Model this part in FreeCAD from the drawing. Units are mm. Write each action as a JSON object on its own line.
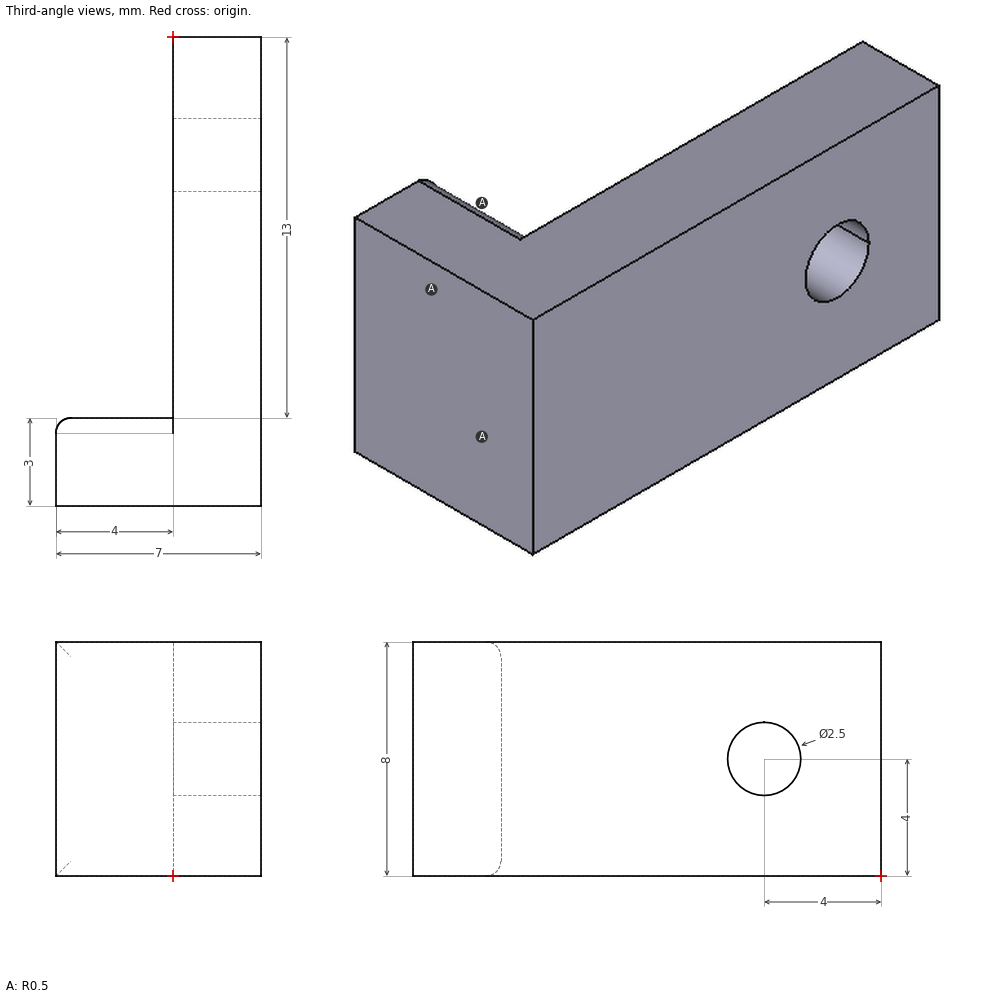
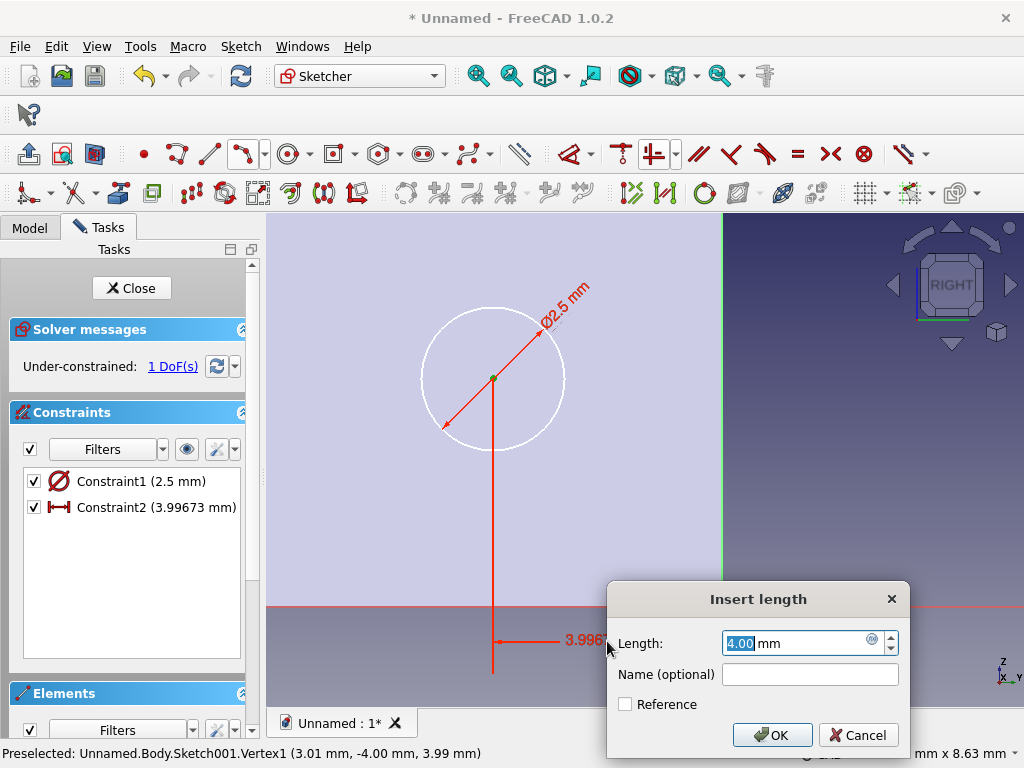
{"action": "type", "text": "4"}
{"action": "key", "text": "Return"}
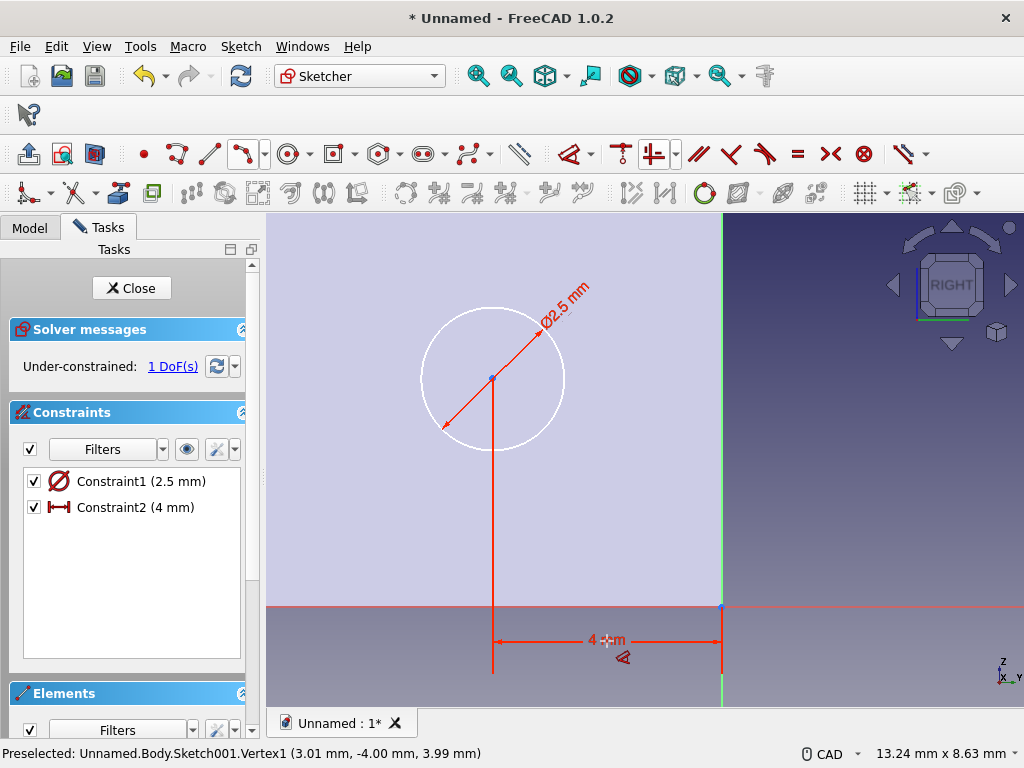
{"action": "left_click", "coordinate": [493, 379]}
{"action": "left_click", "coordinate": [756, 493]}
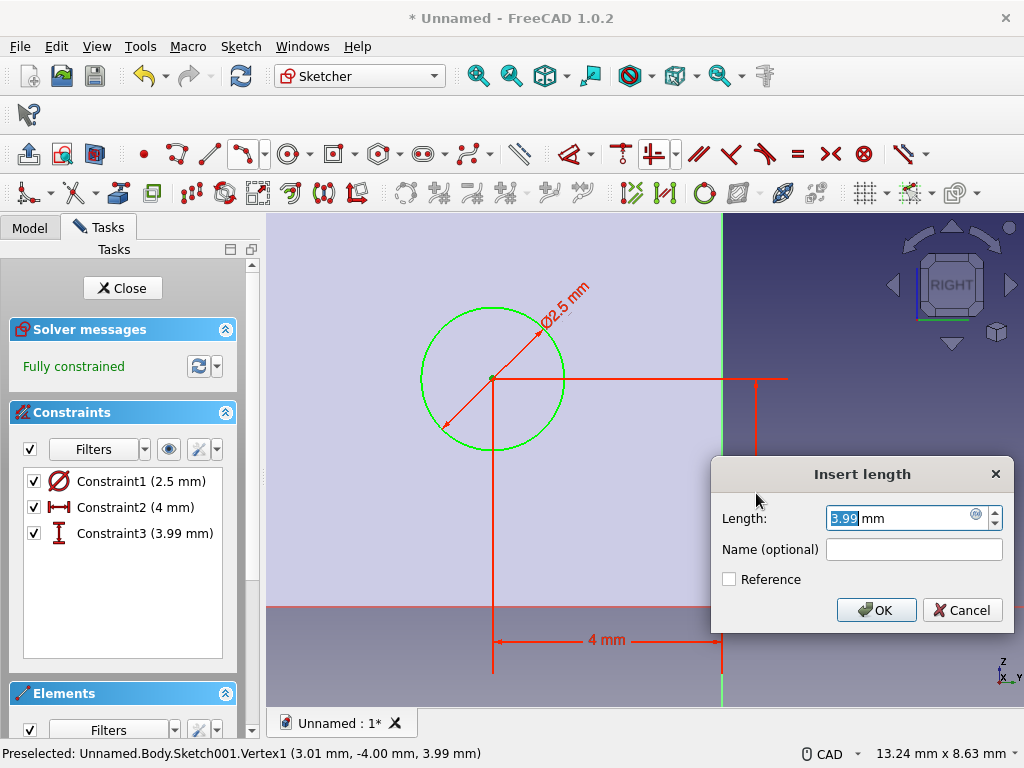
{"action": "type", "text": "4"}
{"action": "key", "text": "Return"}
{"action": "key", "text": "Escape"}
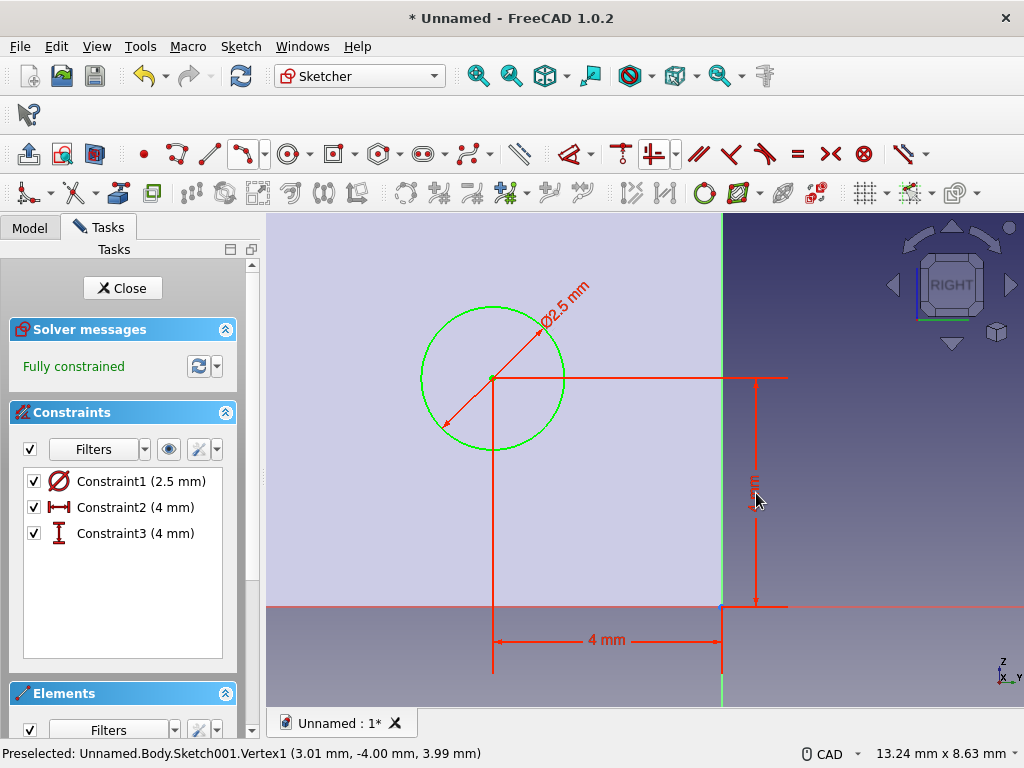
{"action": "left_click", "coordinate": [123, 288]}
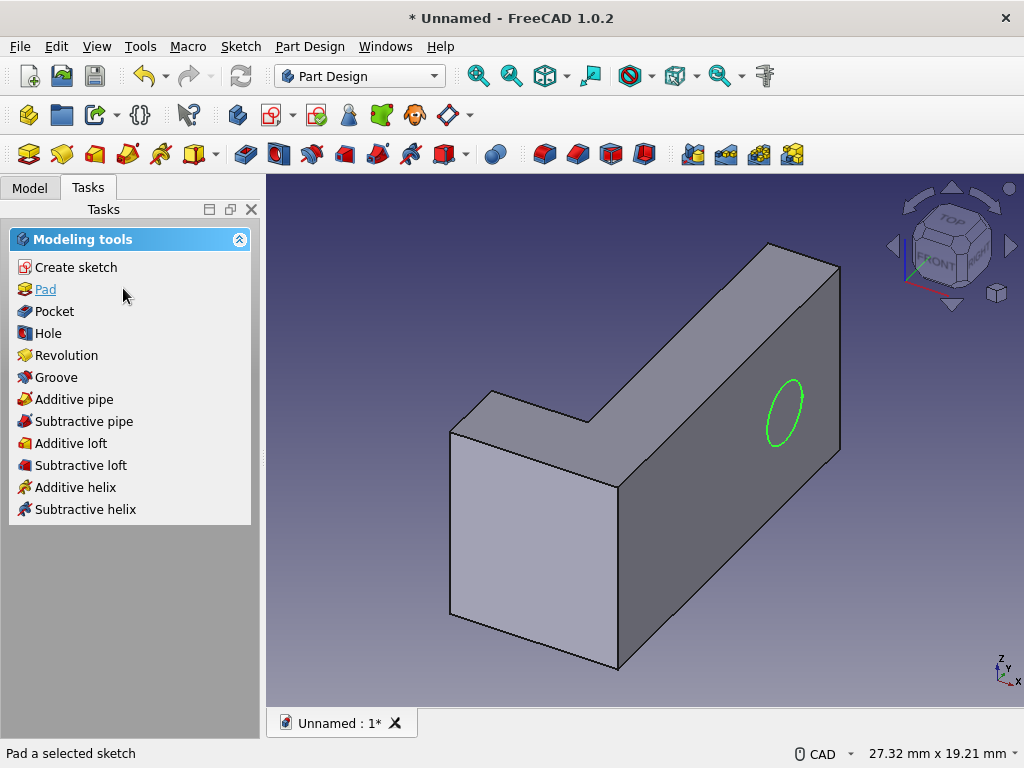
{"action": "left_click", "coordinate": [246, 154]}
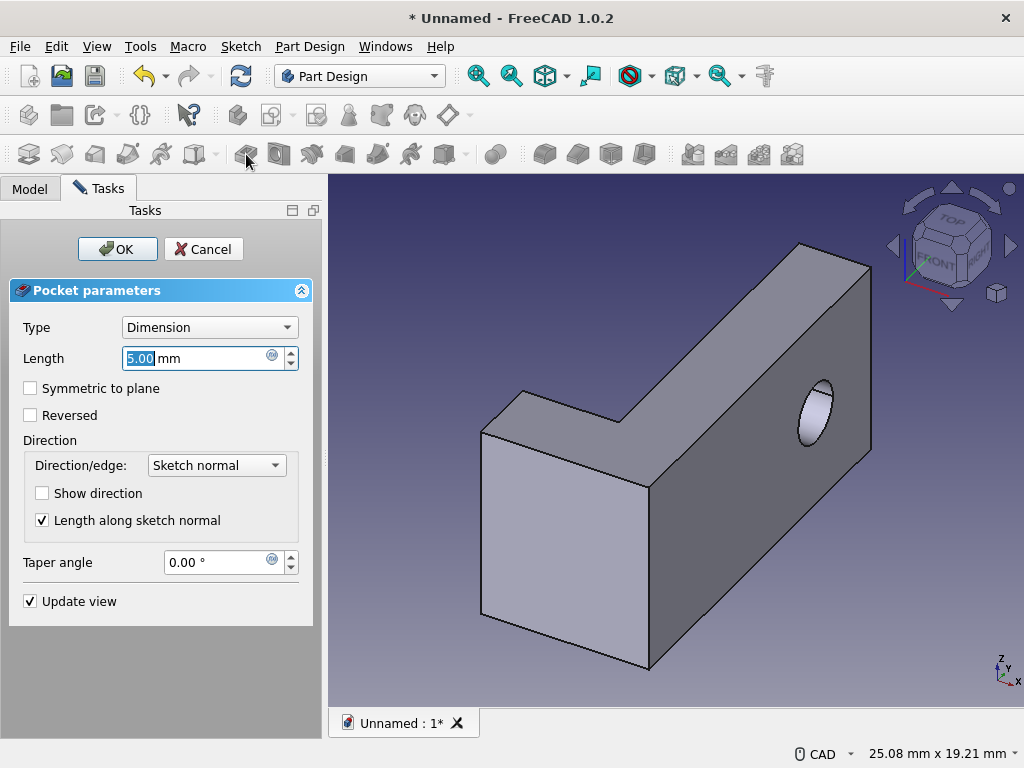
{"action": "left_click", "coordinate": [210, 328]}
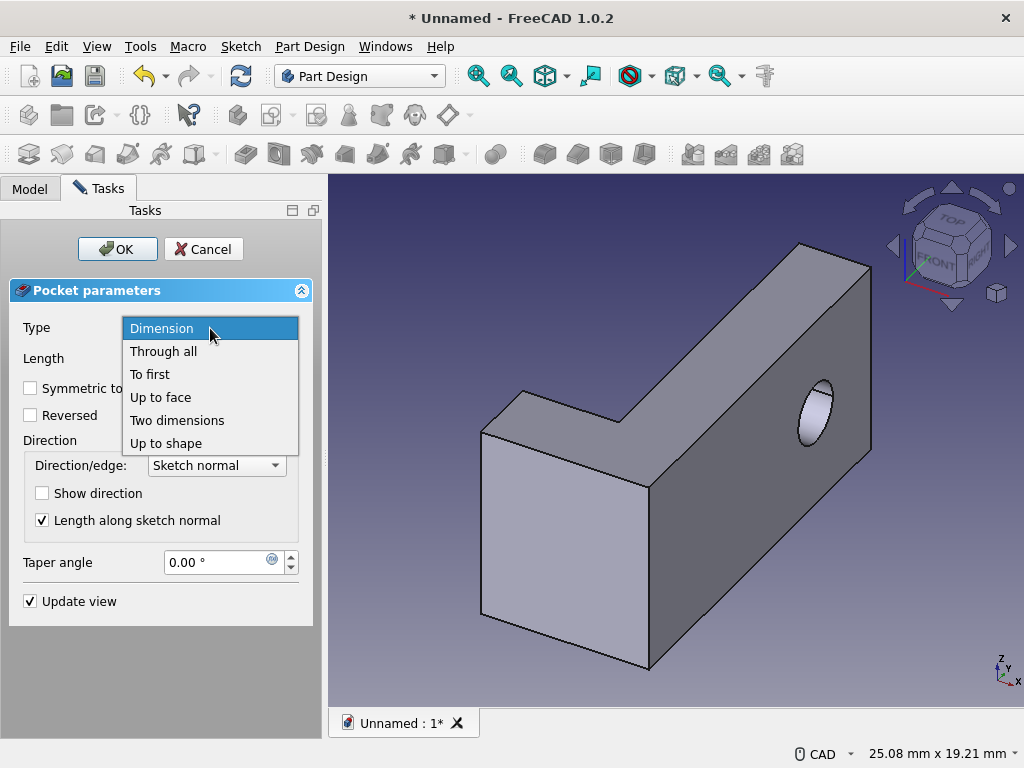
{"action": "left_click", "coordinate": [208, 352]}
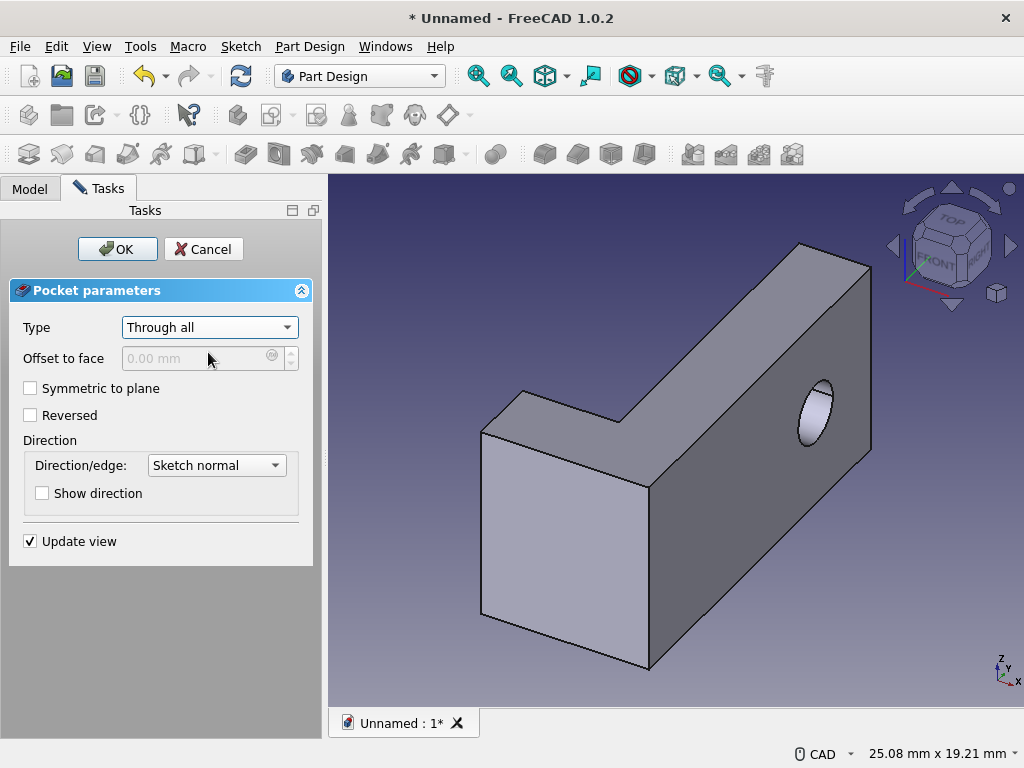
{"action": "left_click", "coordinate": [118, 249]}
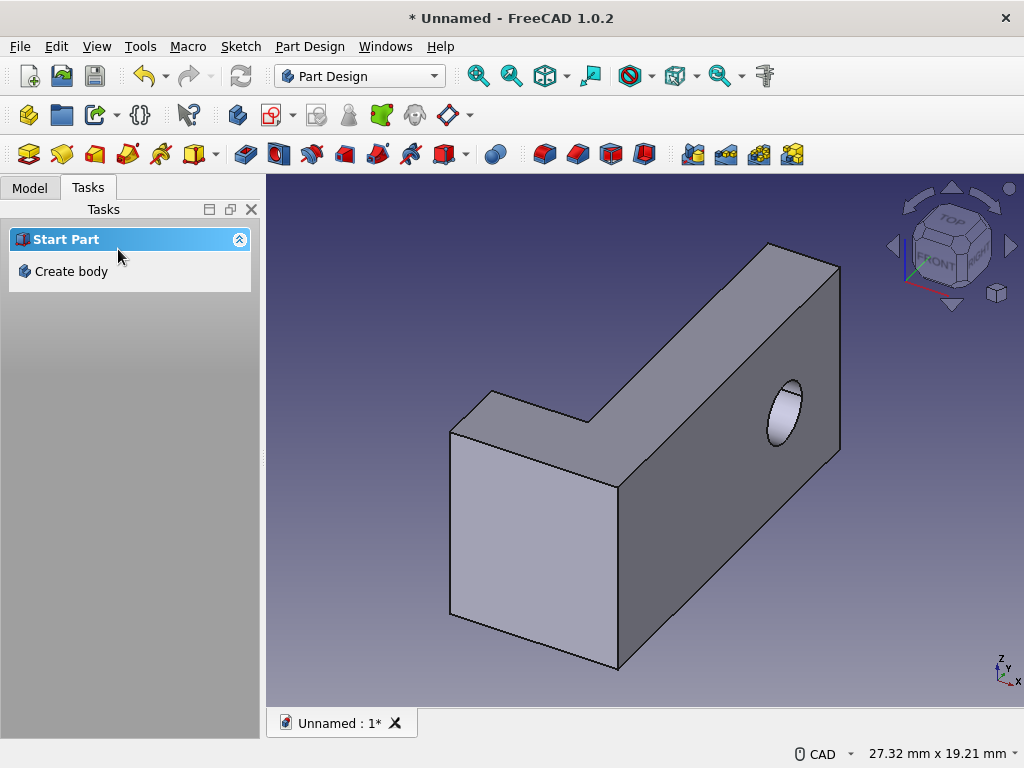
{"action": "key", "text": "0"}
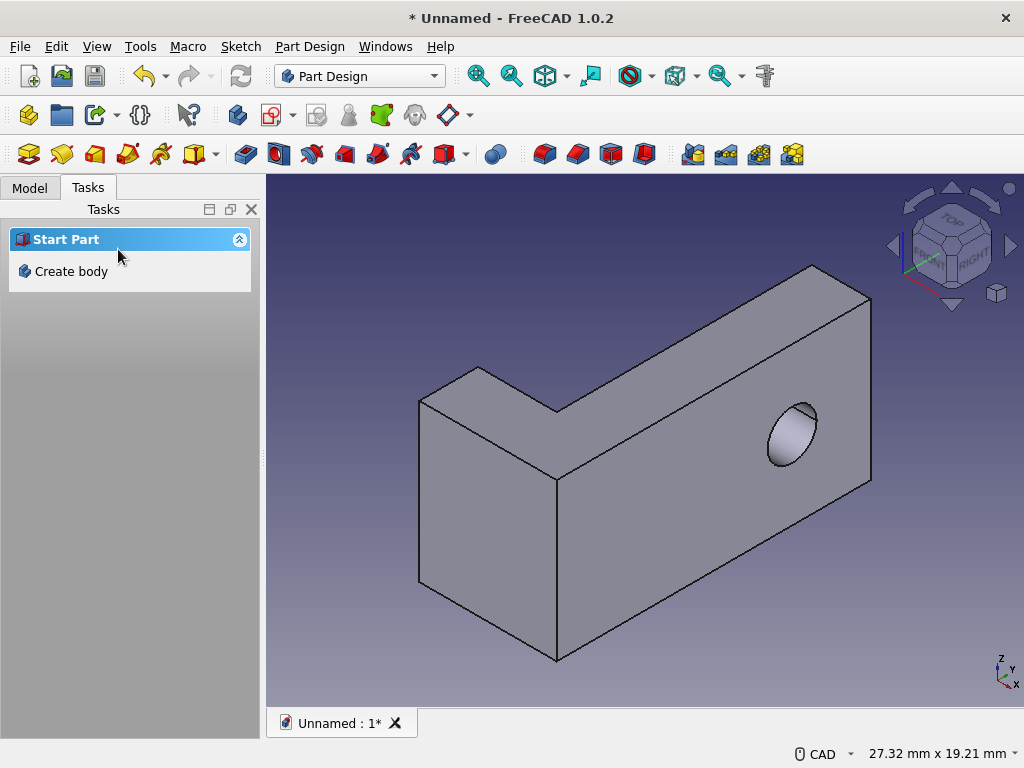
{"action": "key", "text": "2"}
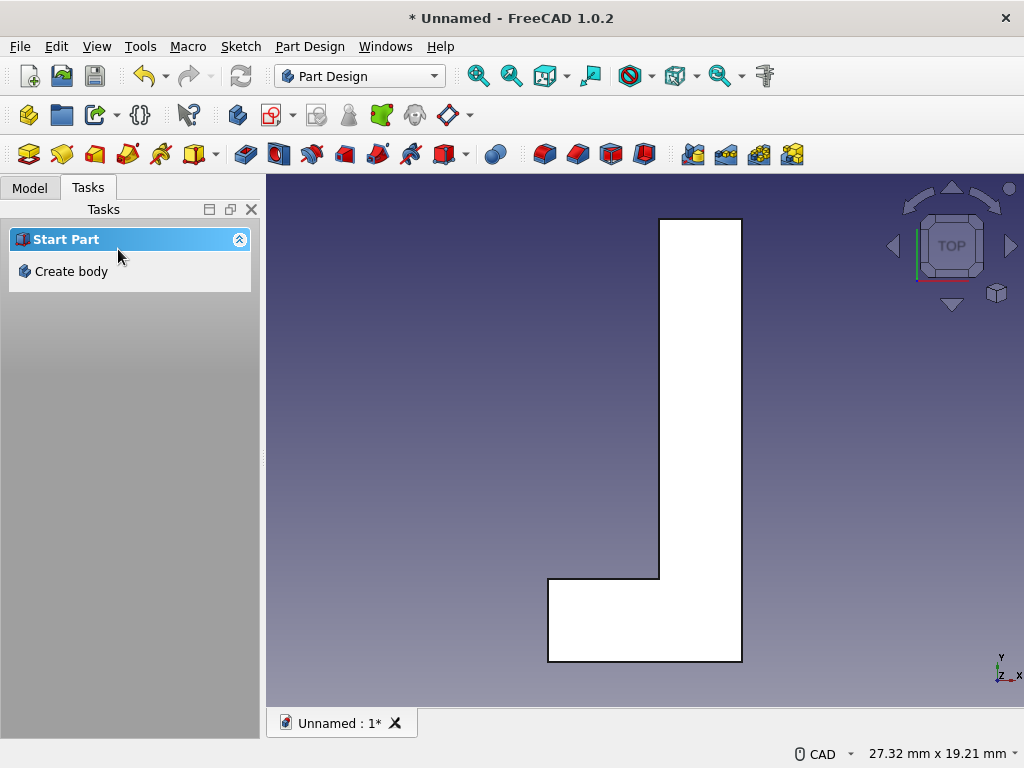
{"action": "left_click", "coordinate": [603, 578]}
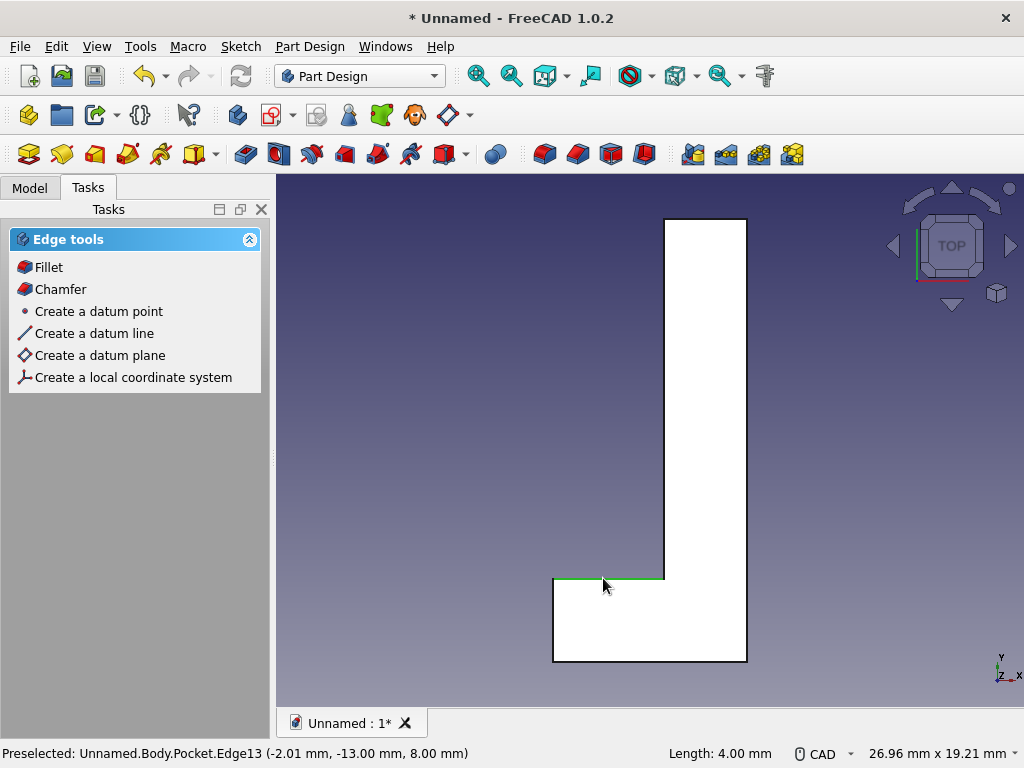
{"action": "key", "text": "1"}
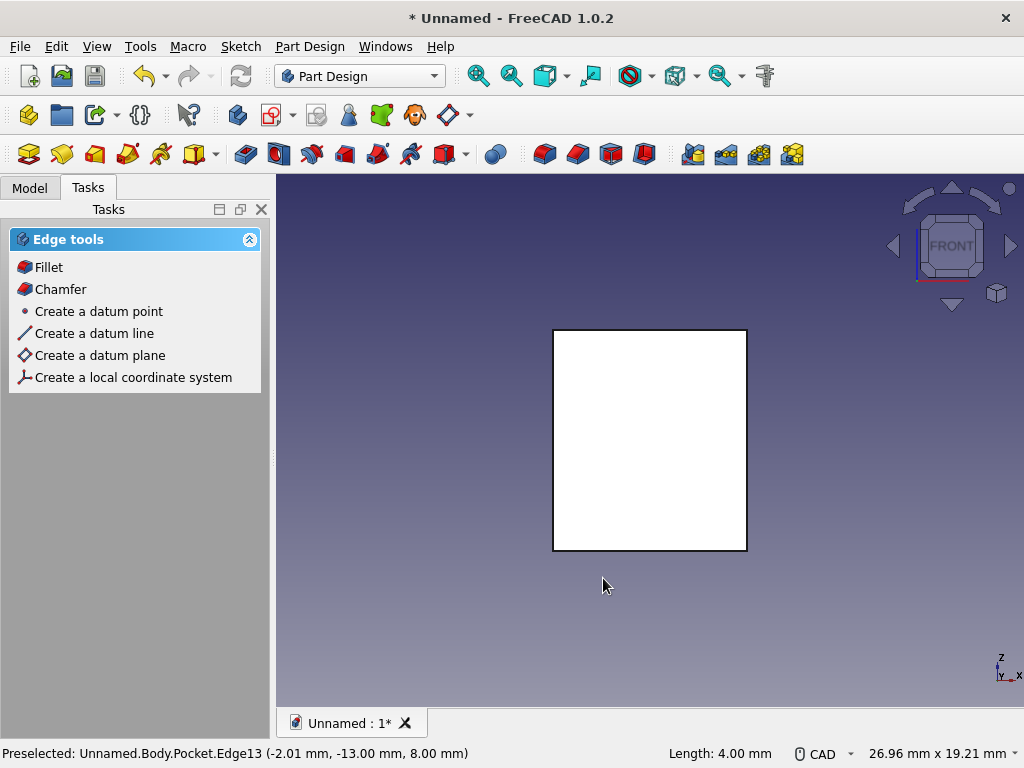
{"action": "key", "text": "v f"}